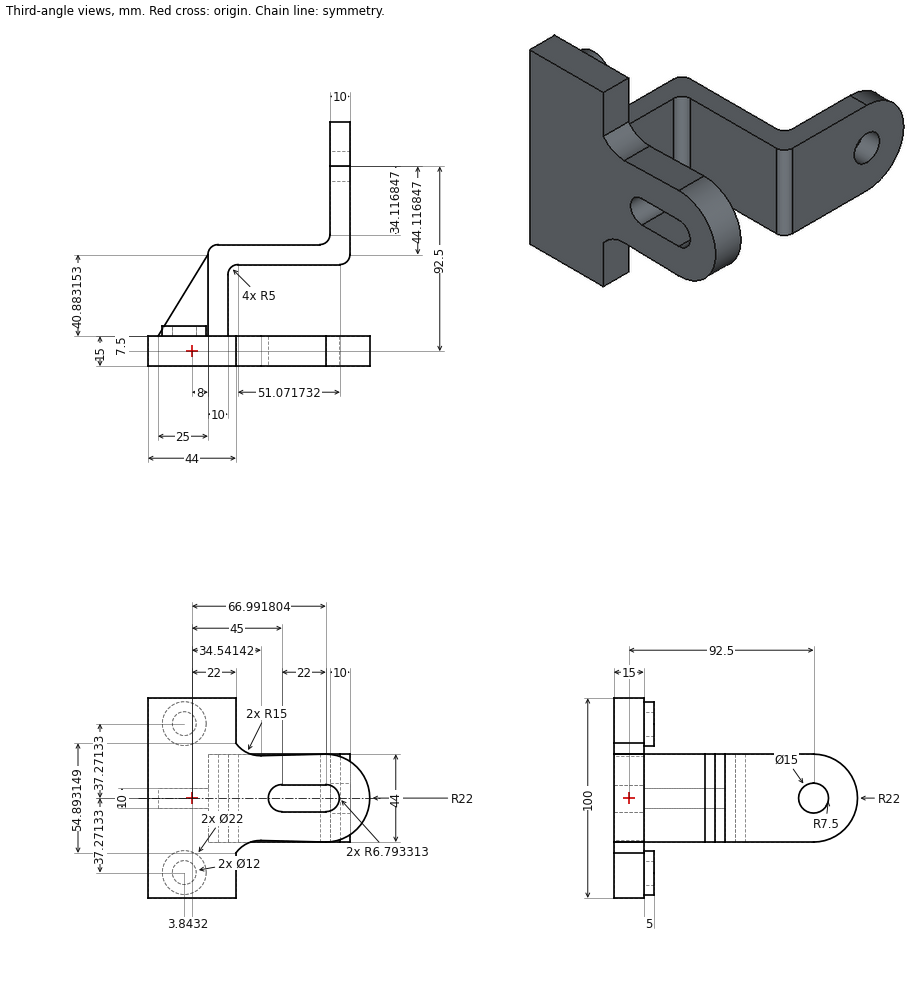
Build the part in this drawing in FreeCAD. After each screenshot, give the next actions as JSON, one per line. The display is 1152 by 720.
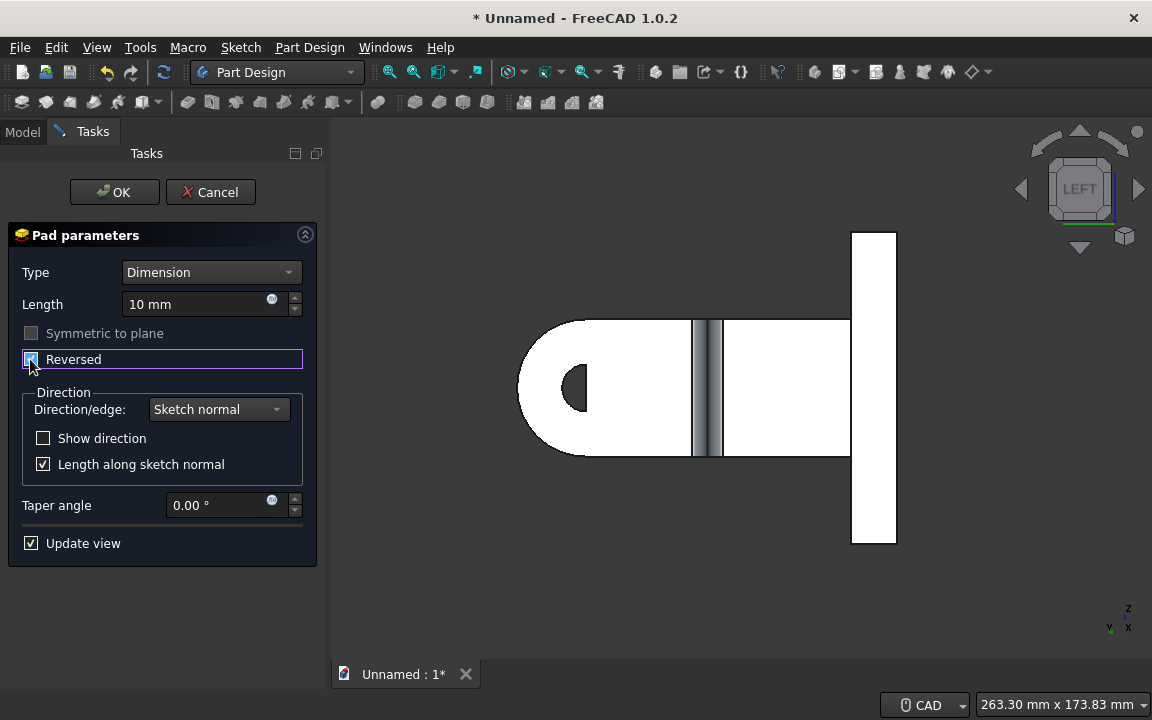
{"action": "left_click", "coordinate": [115, 192]}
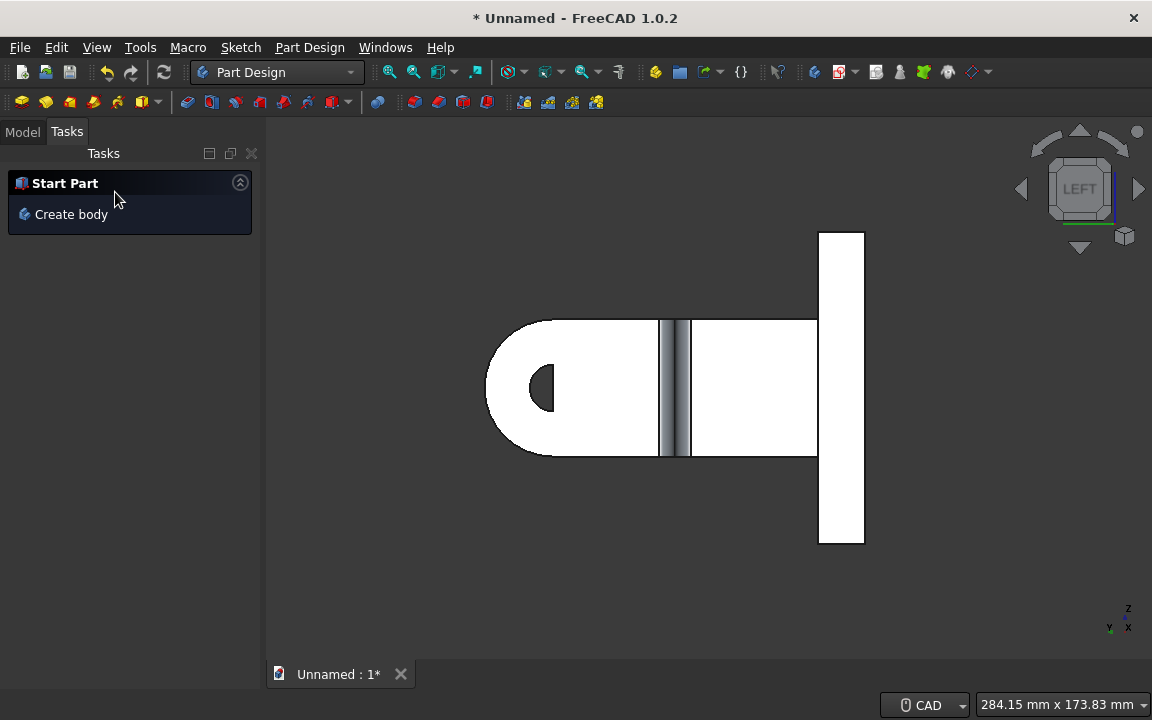
{"action": "left_click", "coordinate": [597, 367]}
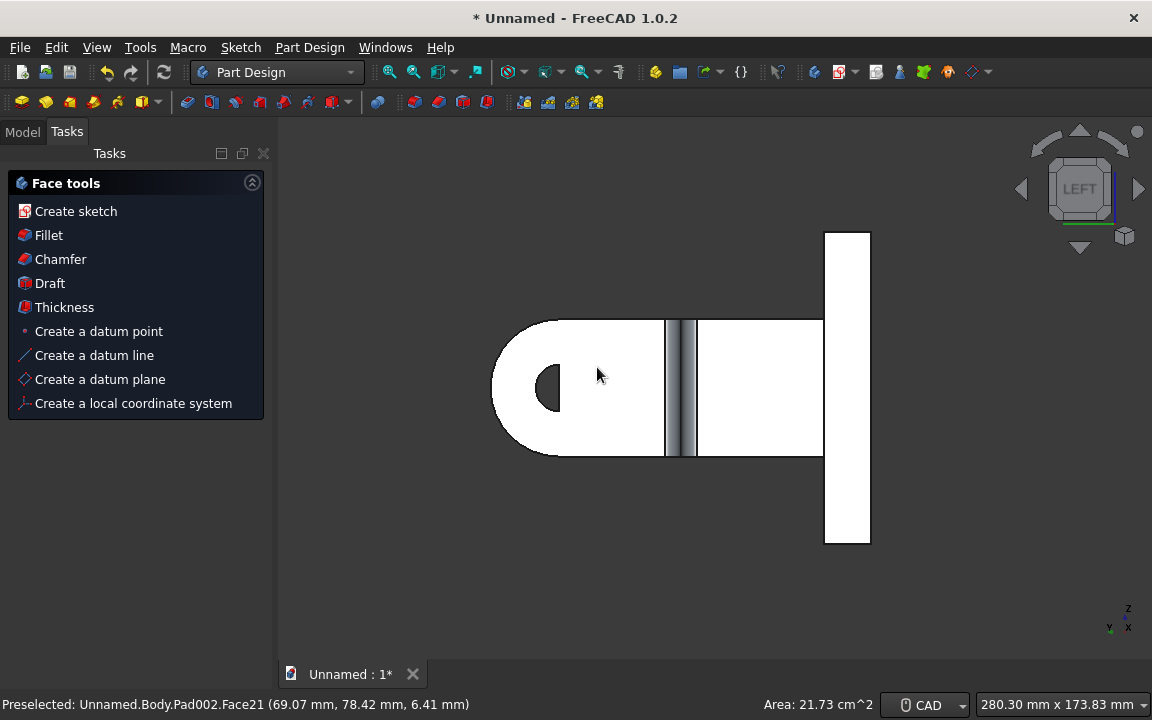
{"action": "left_click", "coordinate": [840, 72]}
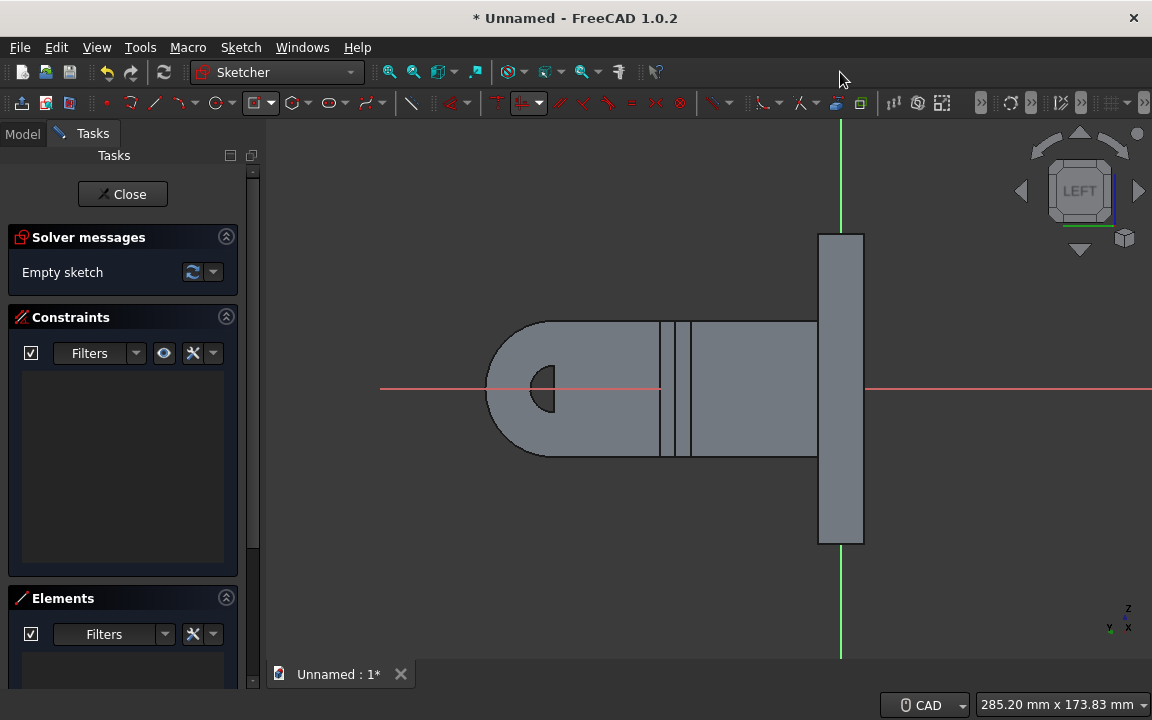
{"action": "left_click", "coordinate": [70, 104]}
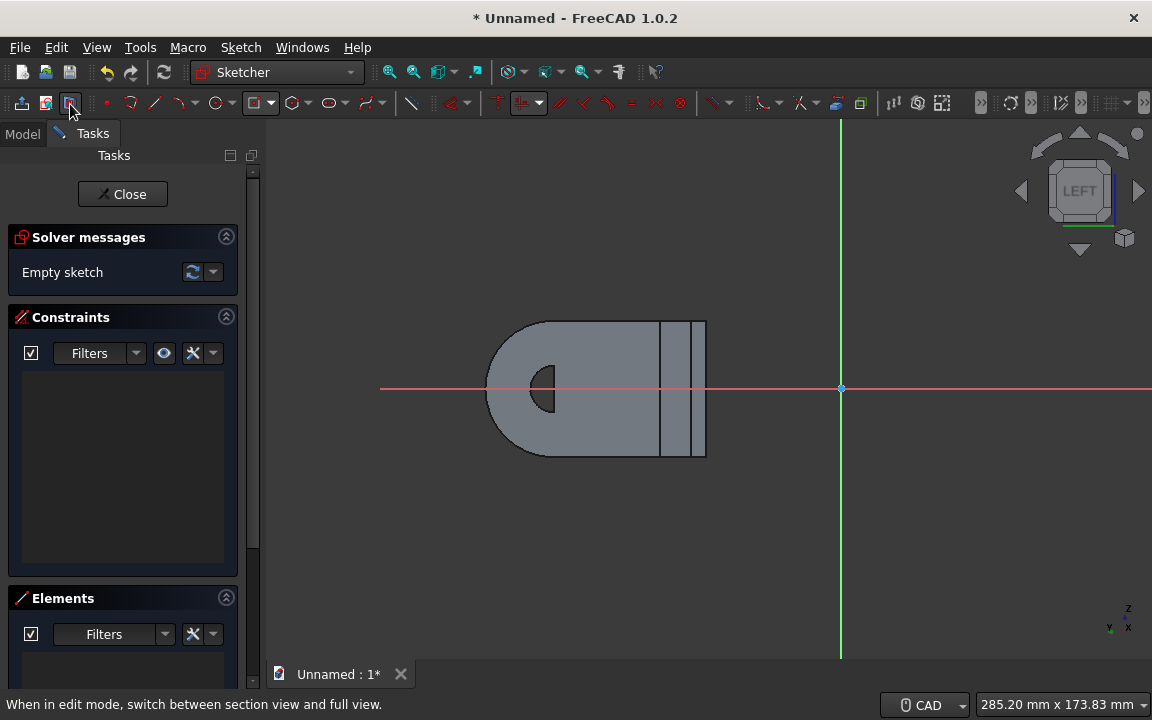
{"action": "scroll", "coordinate": [540, 389], "scroll_direction": "up", "scroll_amount": 10}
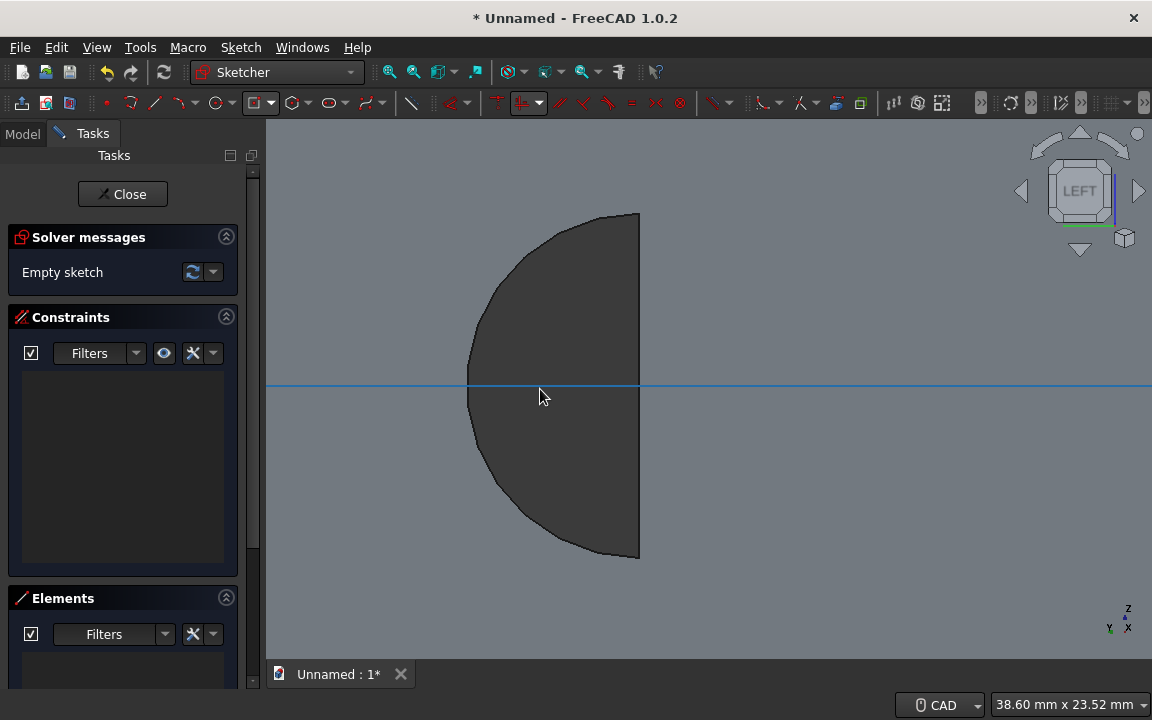
{"action": "left_click", "coordinate": [216, 104]}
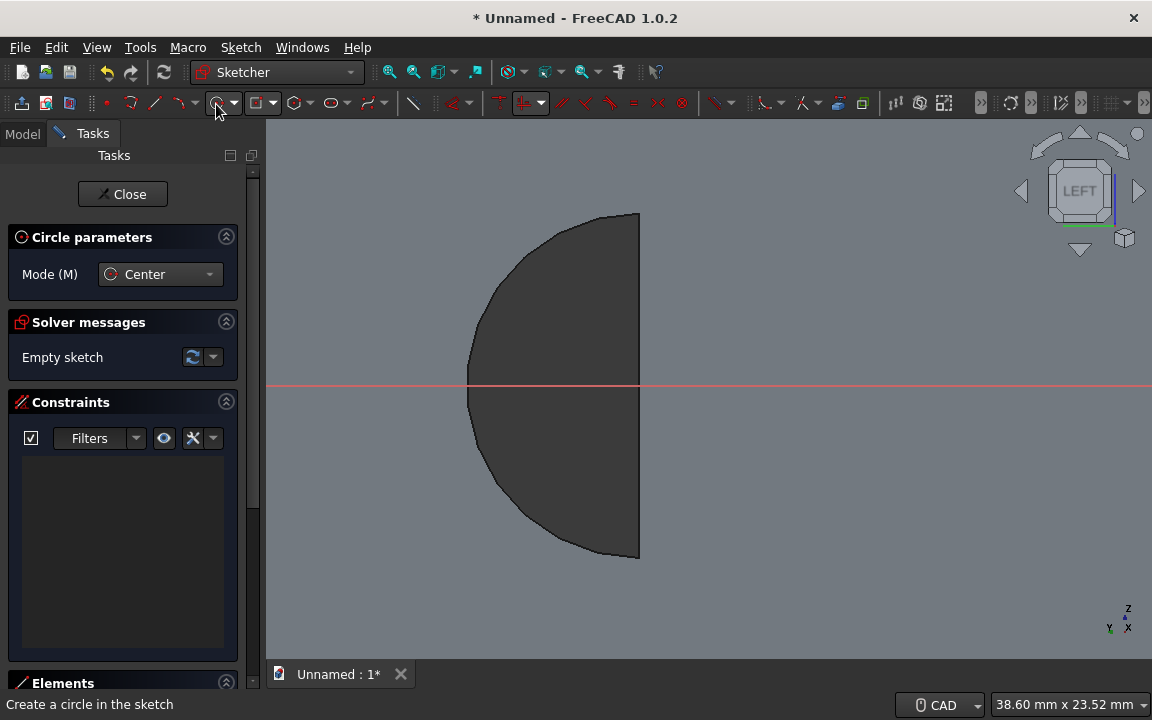
{"action": "left_click", "coordinate": [639, 386]}
{"action": "mouse_move", "coordinate": [761, 264]}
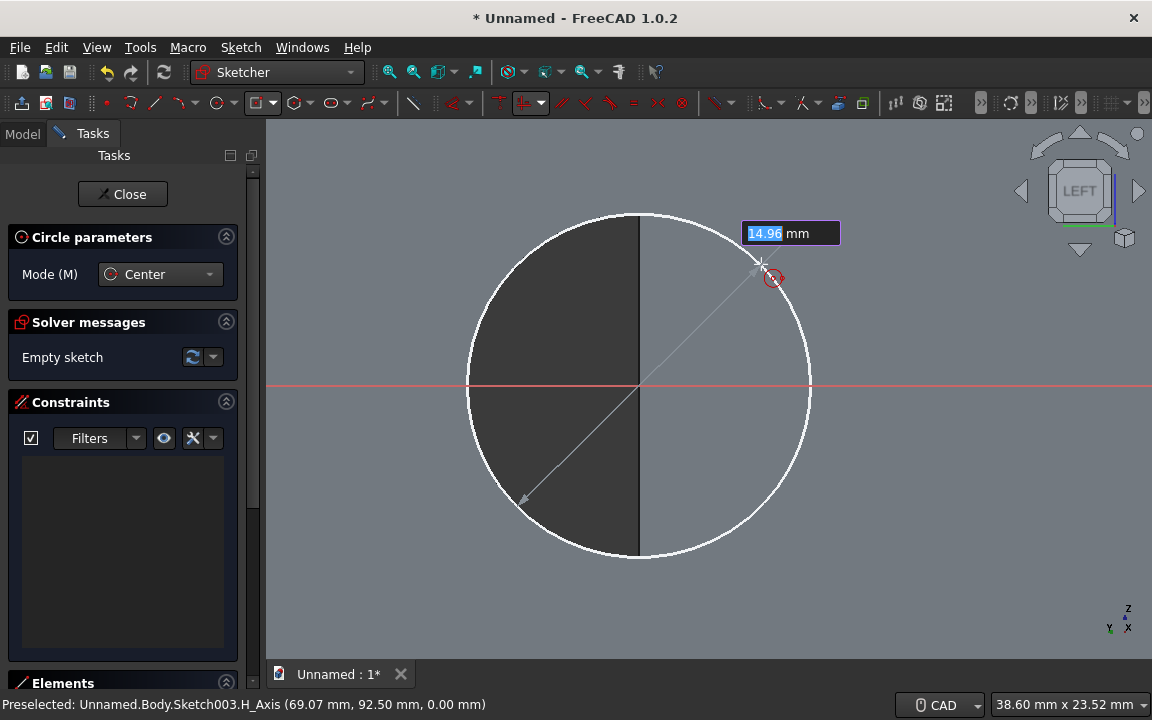
{"action": "type", "text": "15"}
{"action": "key", "text": "Return"}
{"action": "key", "text": "Escape"}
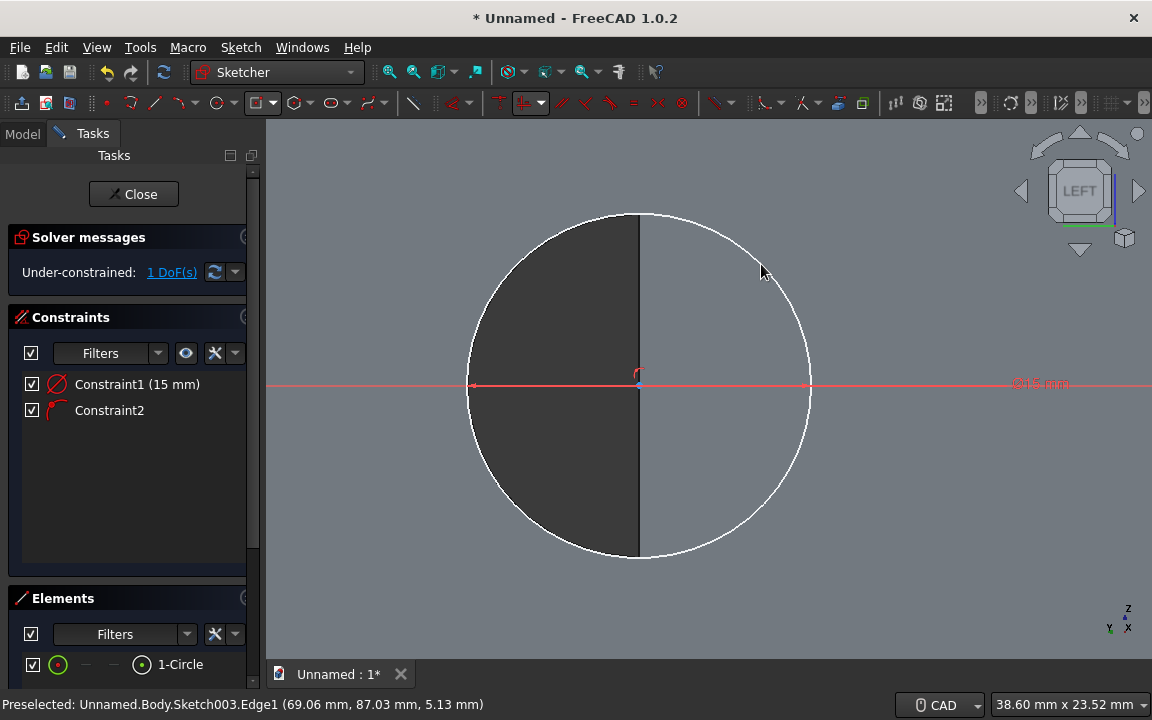
{"action": "left_click", "coordinate": [452, 104]}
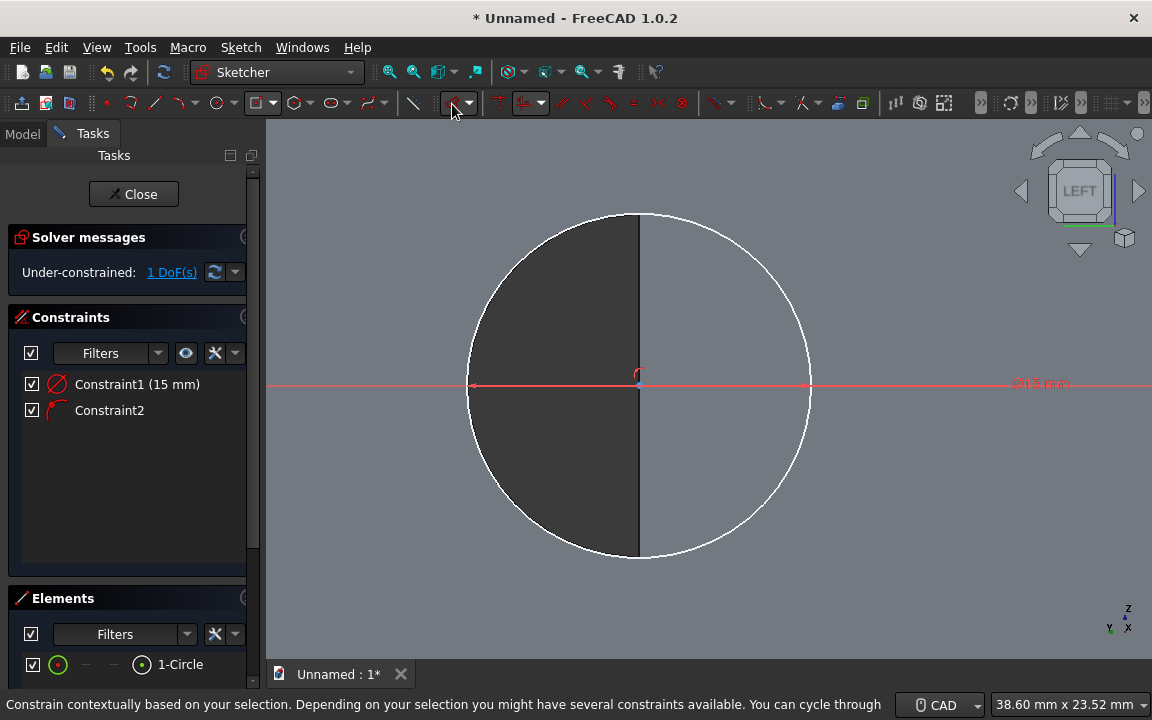
{"action": "left_click", "coordinate": [639, 386]}
{"action": "left_click", "coordinate": [733, 420]}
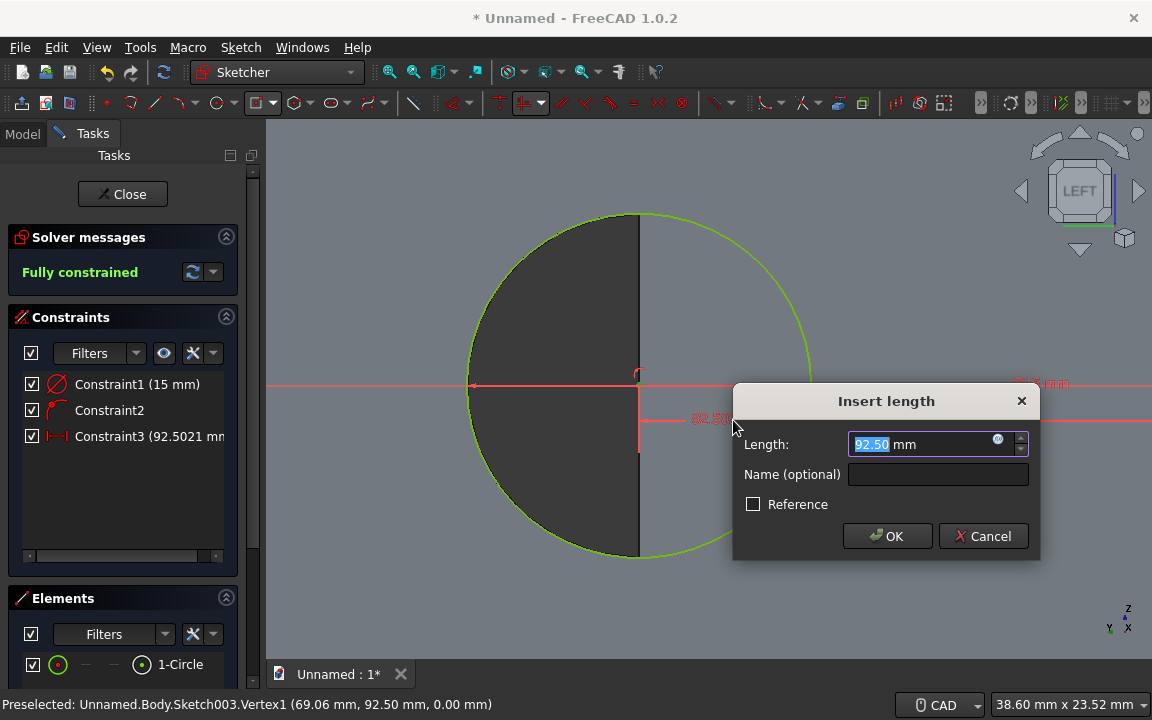
{"action": "type", "text": "92.5"}
{"action": "key", "text": "Return"}
{"action": "key", "text": "Escape"}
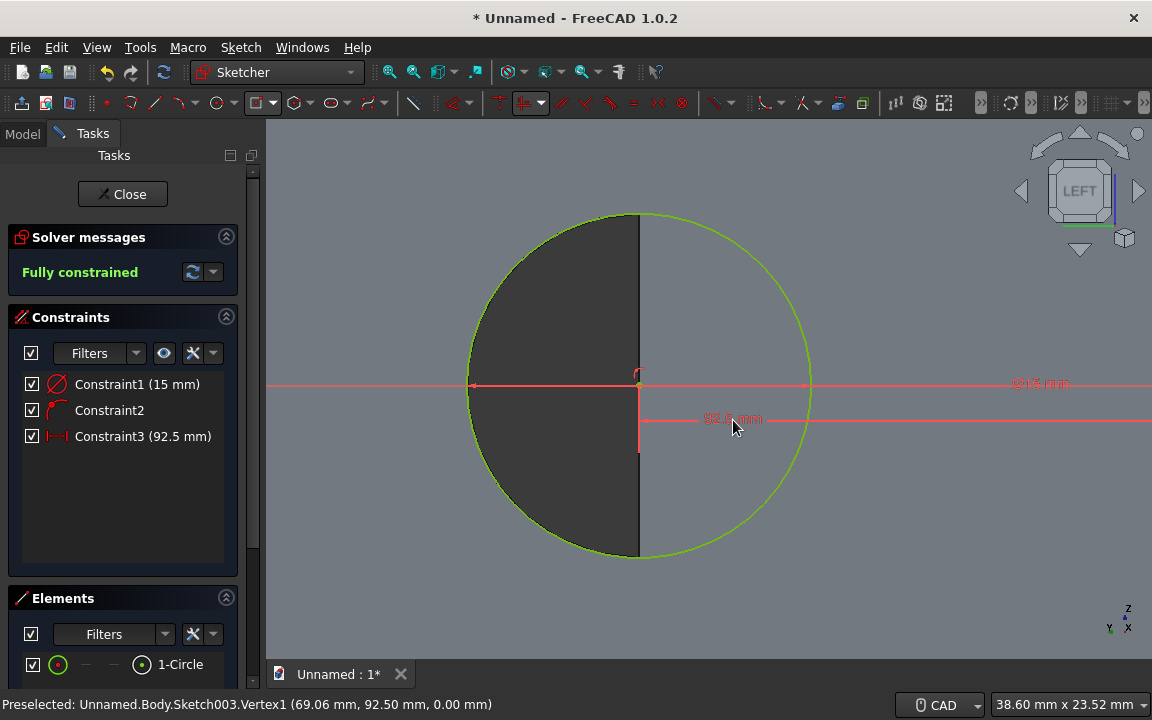
{"action": "left_click", "coordinate": [123, 194]}